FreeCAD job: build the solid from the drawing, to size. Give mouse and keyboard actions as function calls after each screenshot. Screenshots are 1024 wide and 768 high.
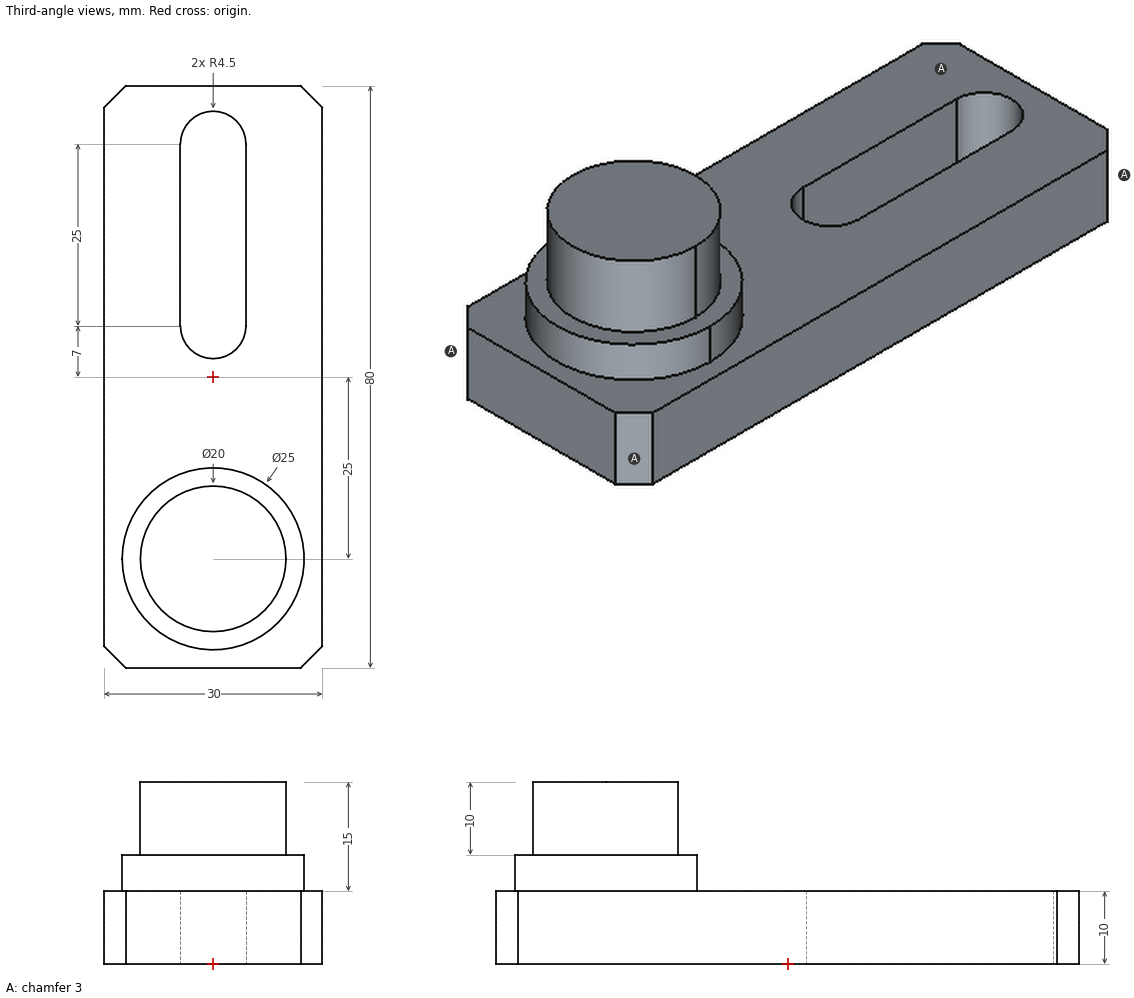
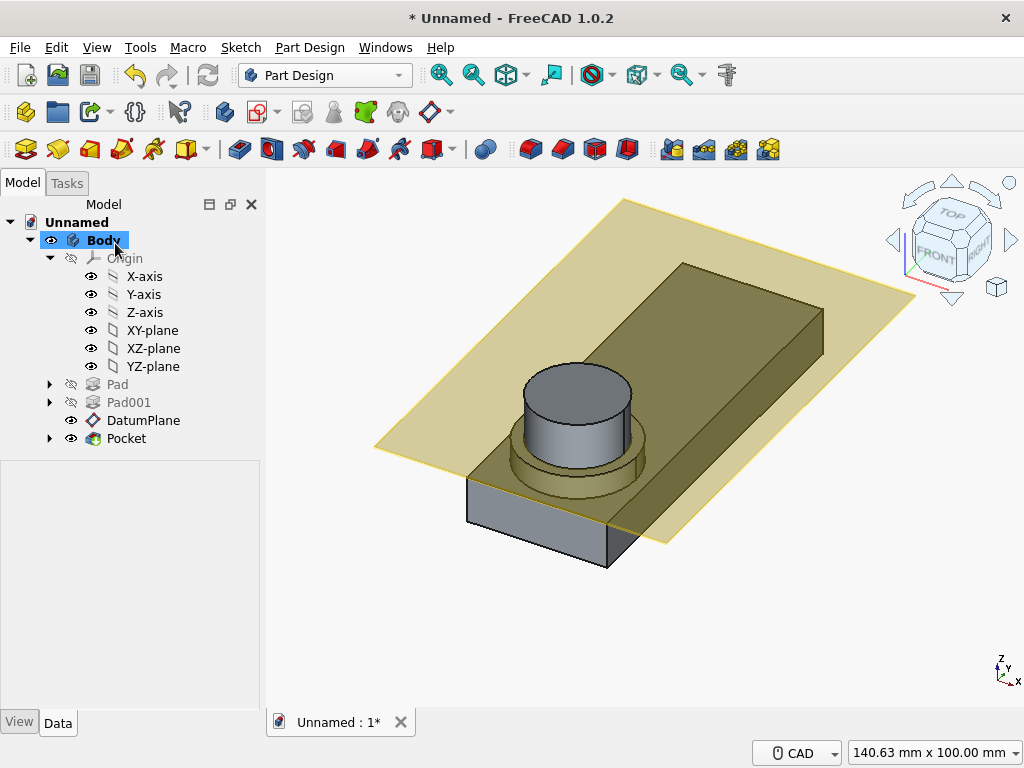
click(116, 420)
key(space)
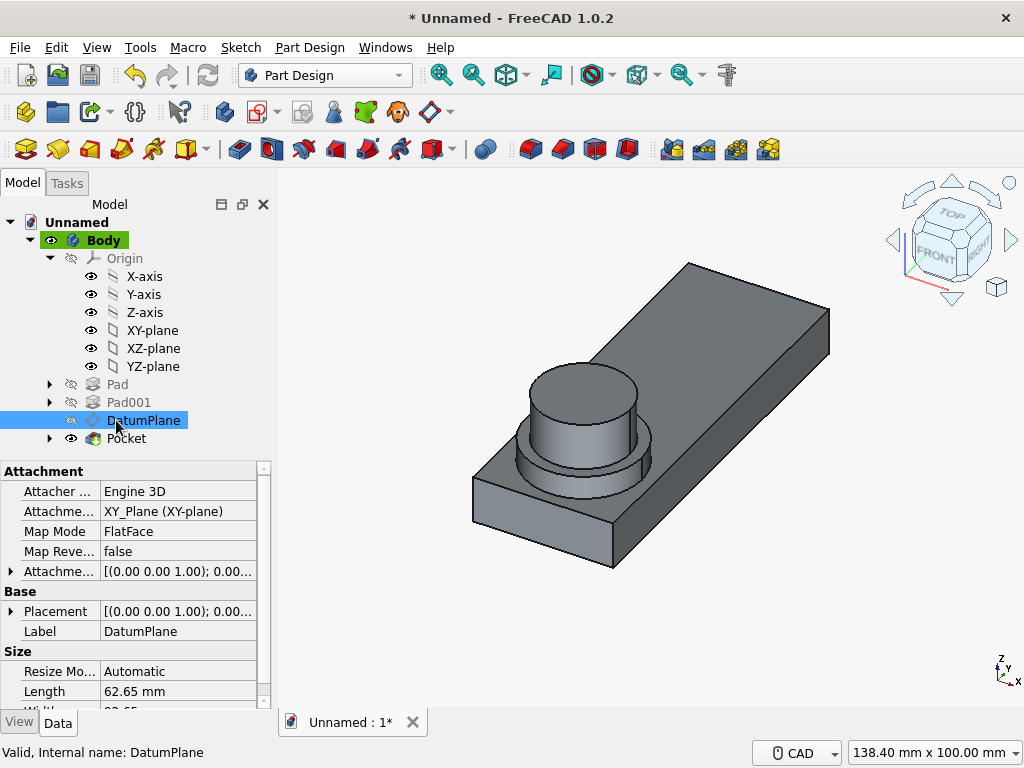
click(713, 331)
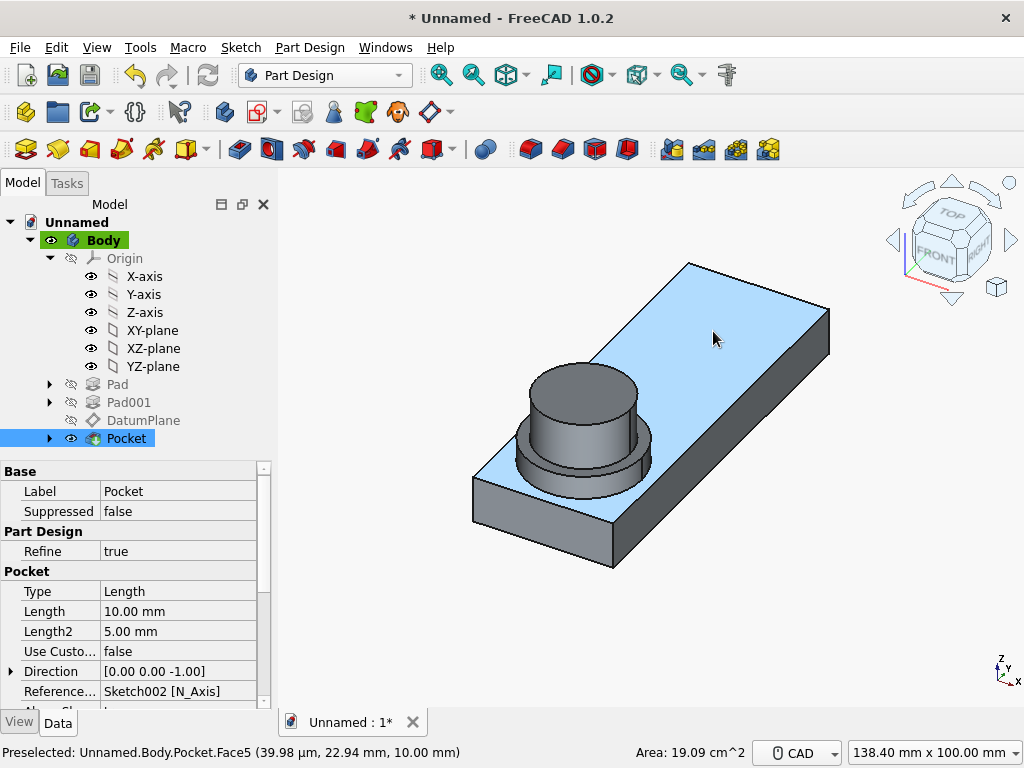
click(258, 112)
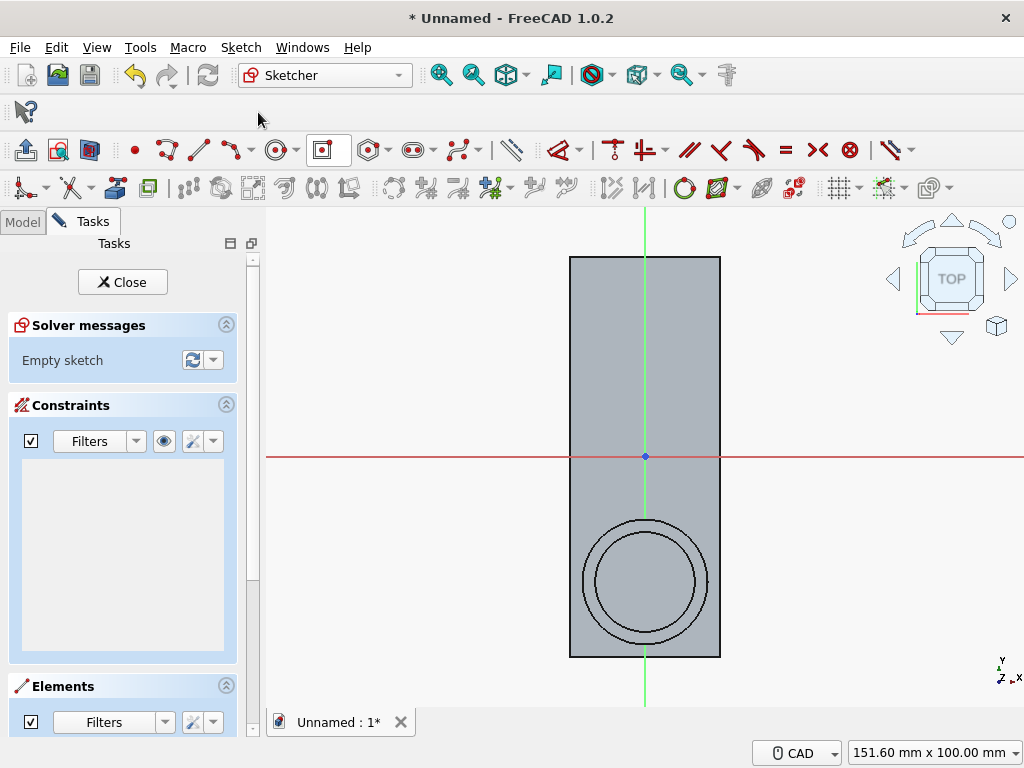
click(90, 150)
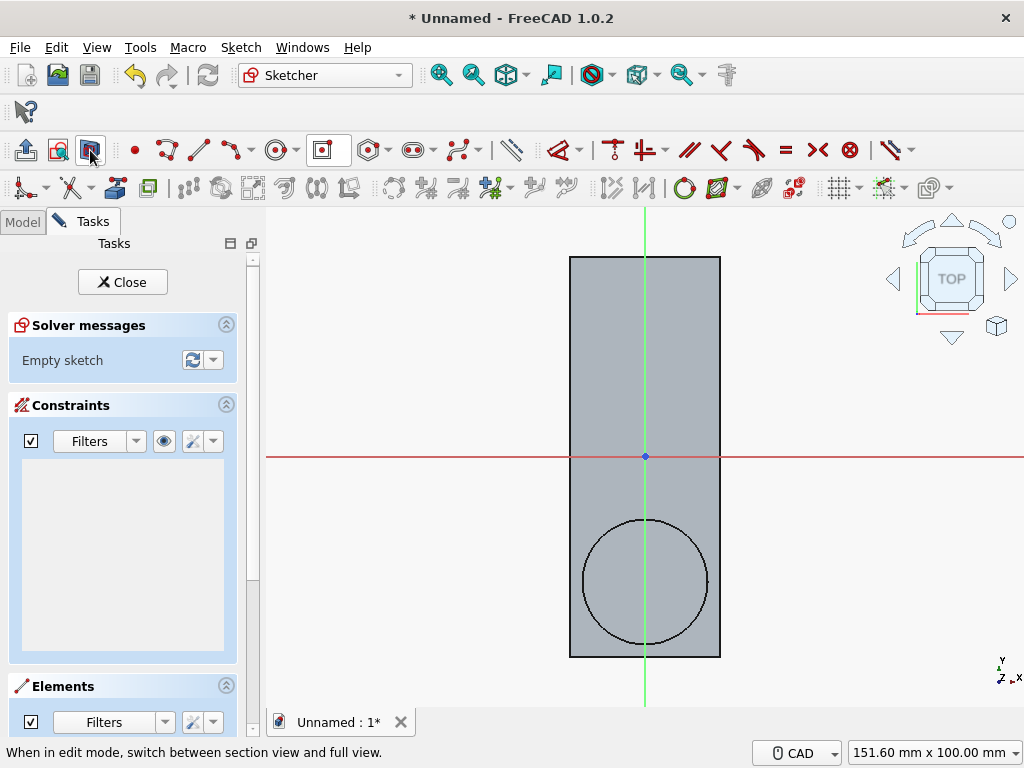
scroll(728, 255, up, 3)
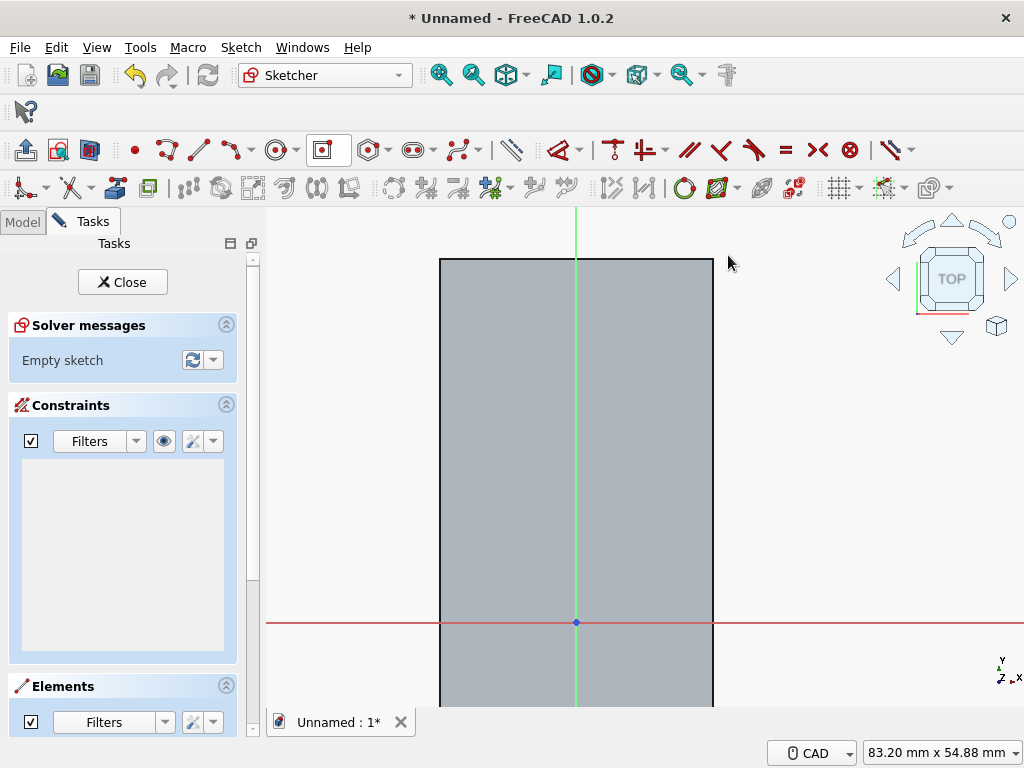
click(414, 150)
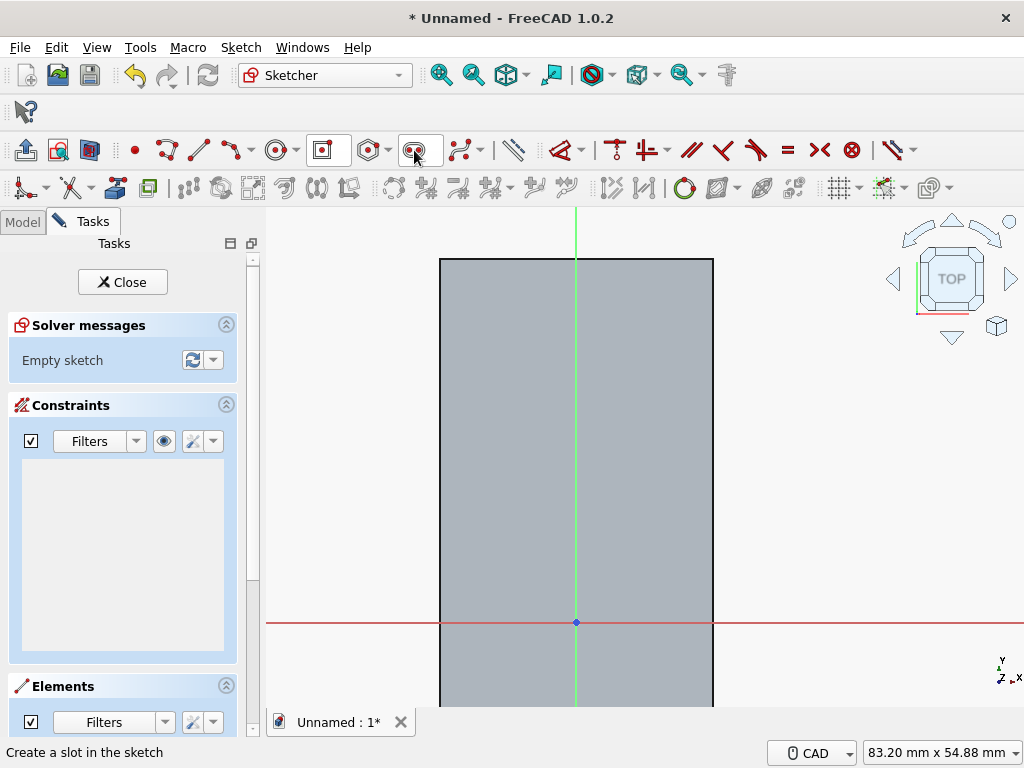
click(576, 559)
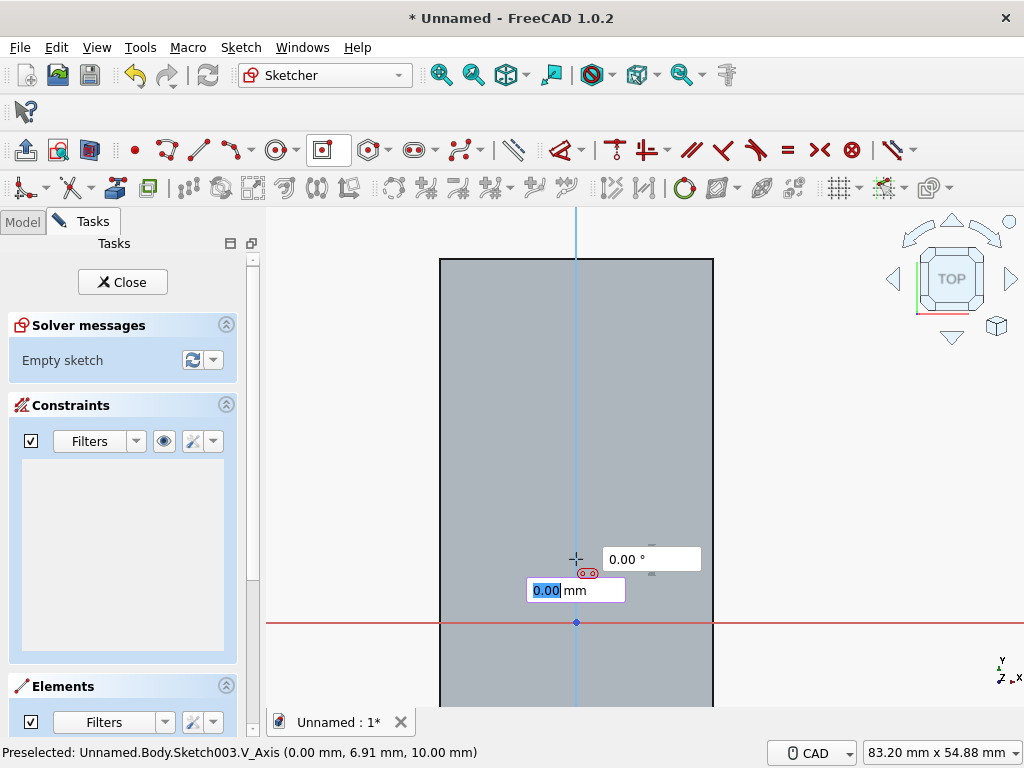
click(585, 331)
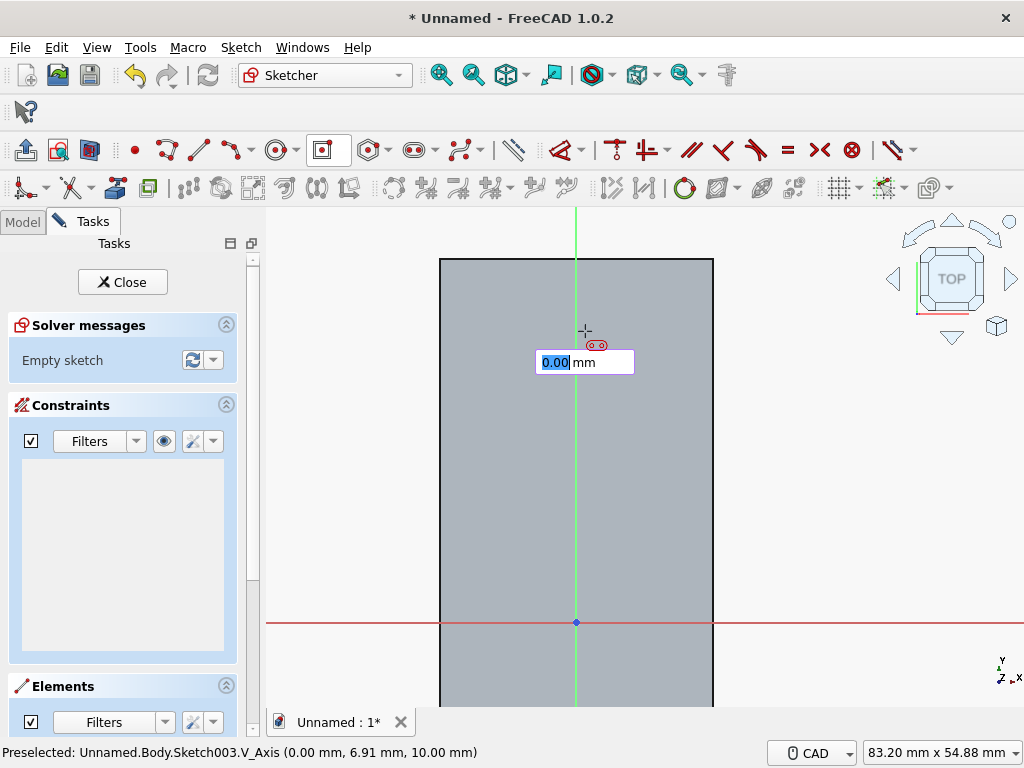
click(617, 445)
key(Escape)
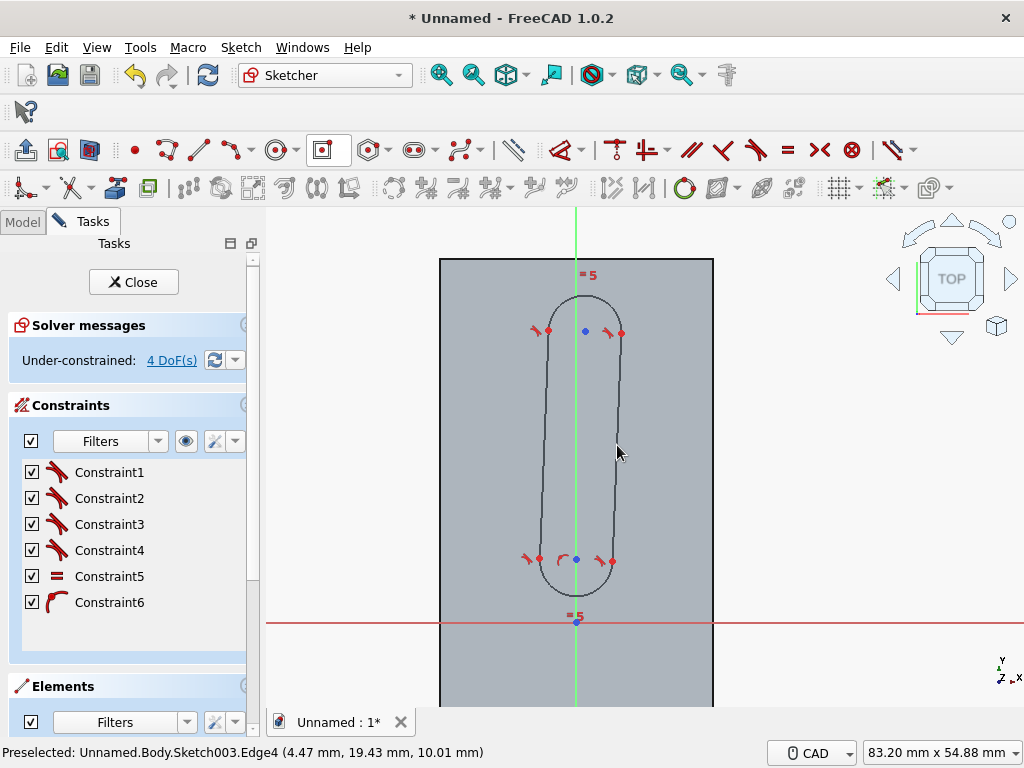
click(543, 490)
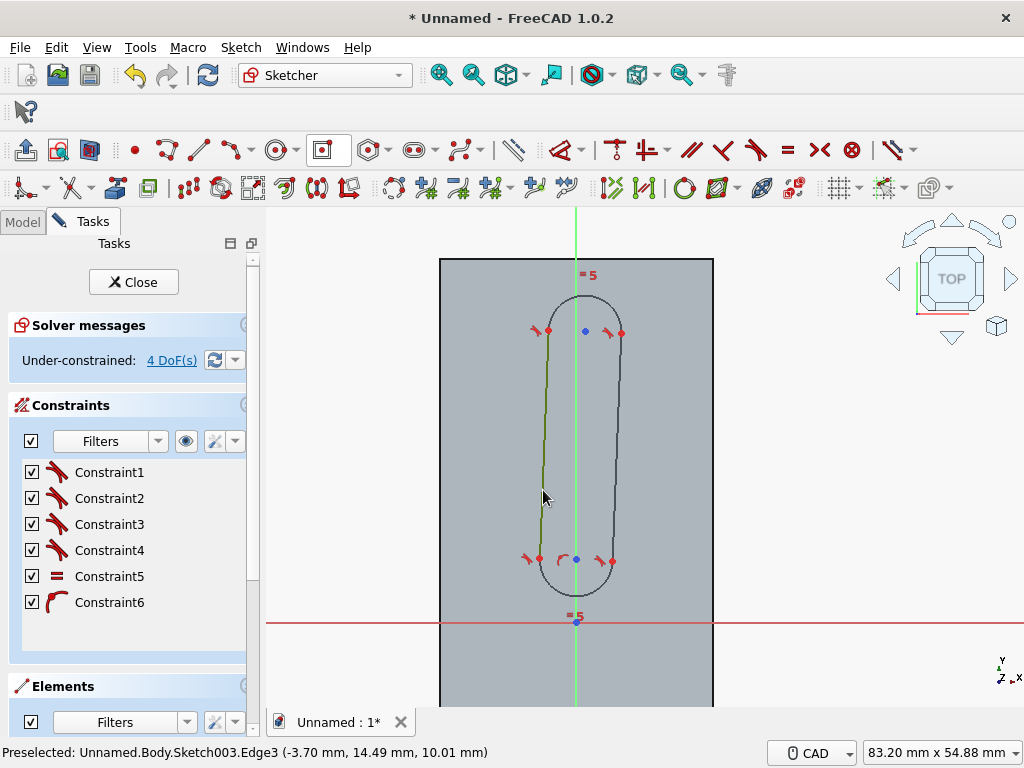
key(v)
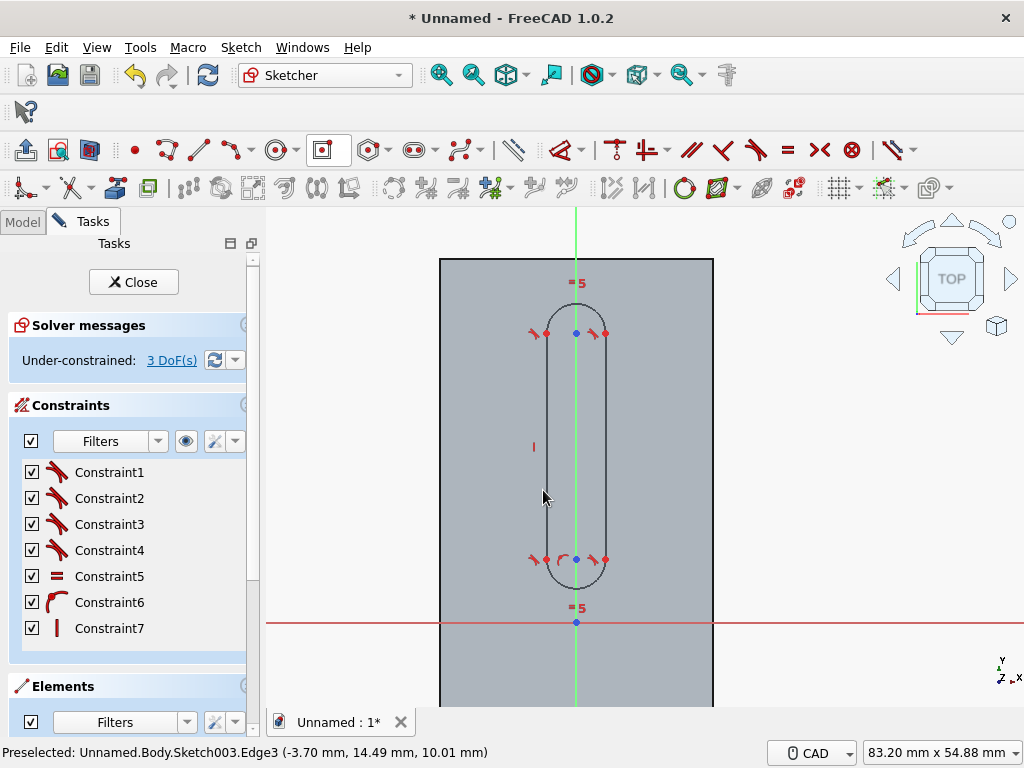
click(560, 150)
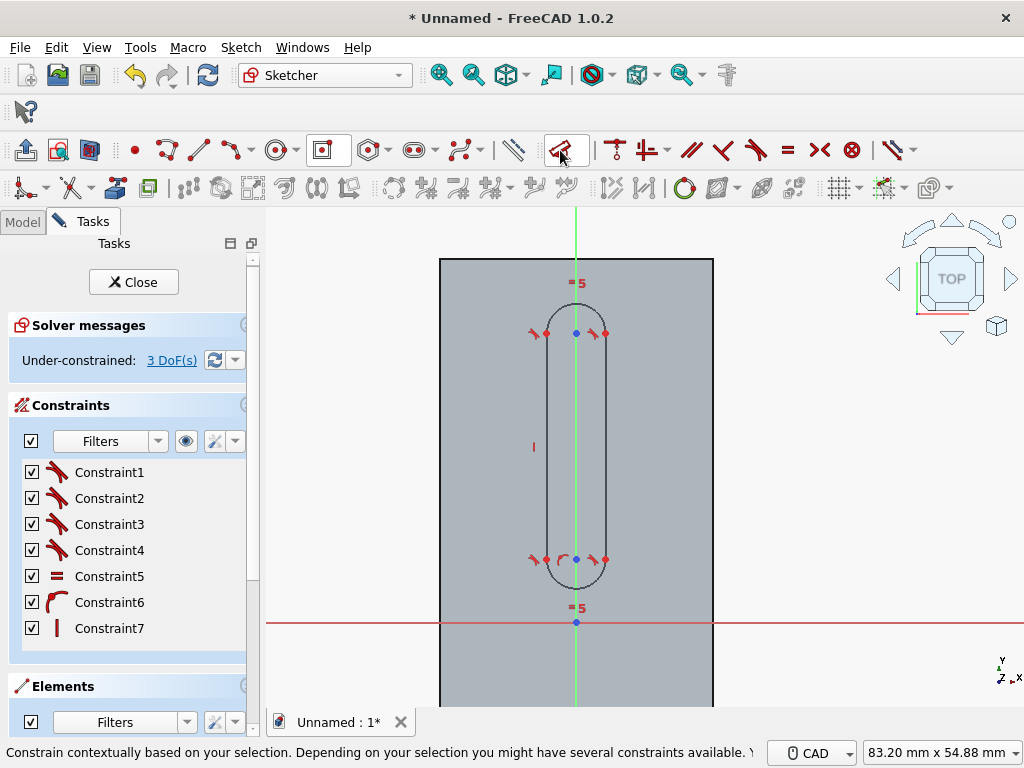
click(559, 583)
click(540, 609)